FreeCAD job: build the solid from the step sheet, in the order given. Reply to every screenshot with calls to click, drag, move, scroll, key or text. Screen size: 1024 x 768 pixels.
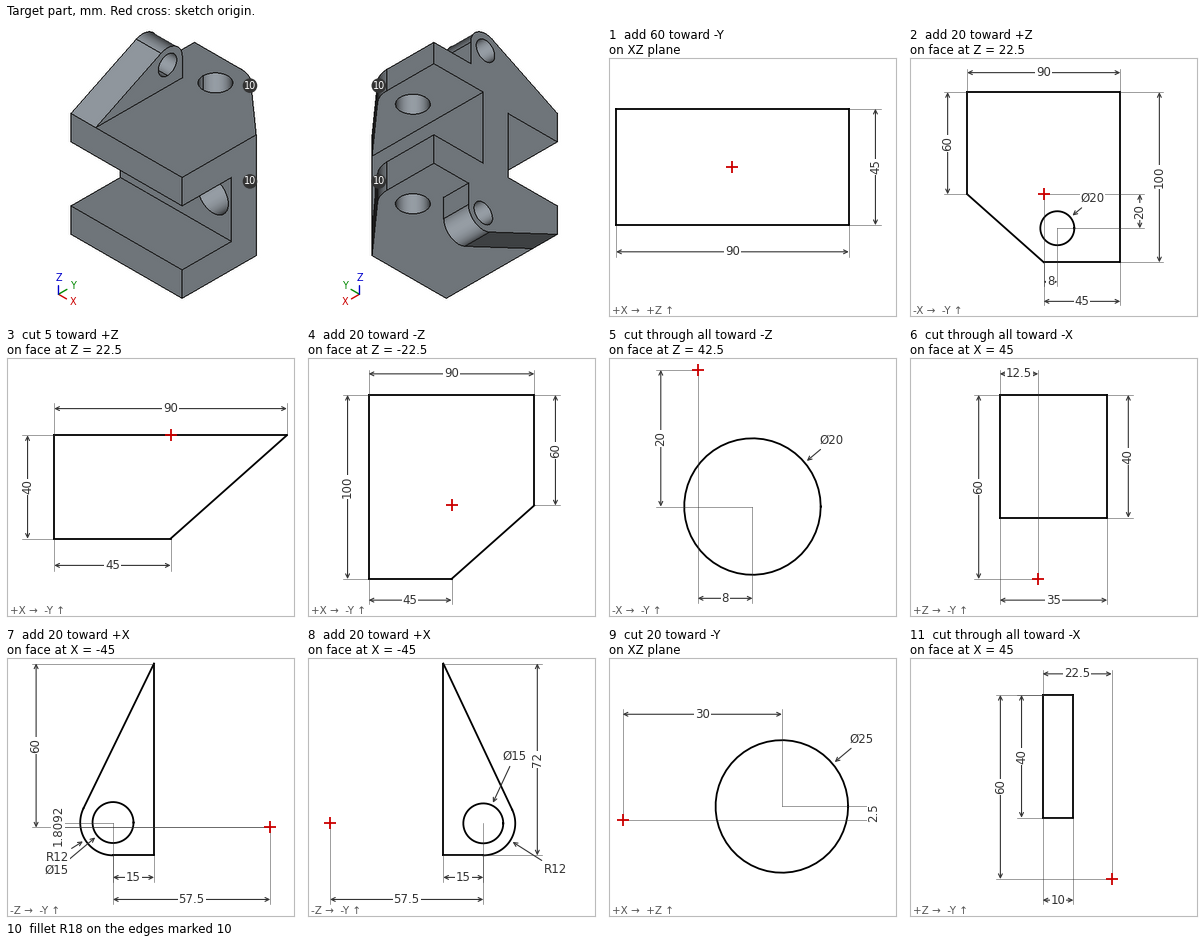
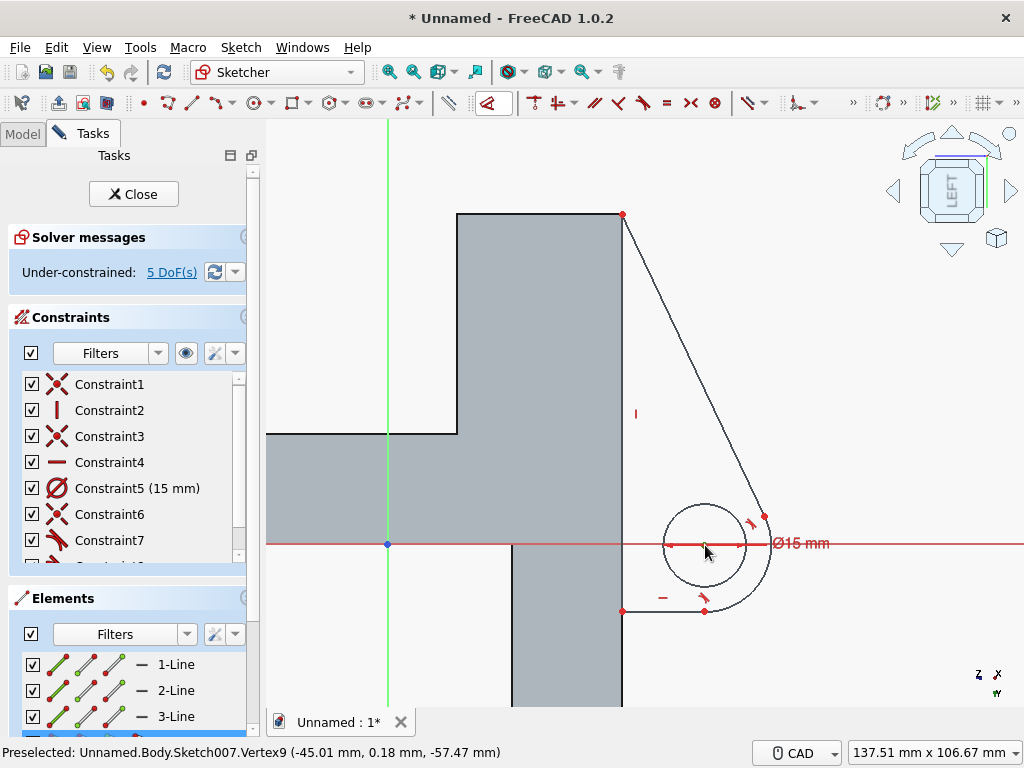
click(334, 544)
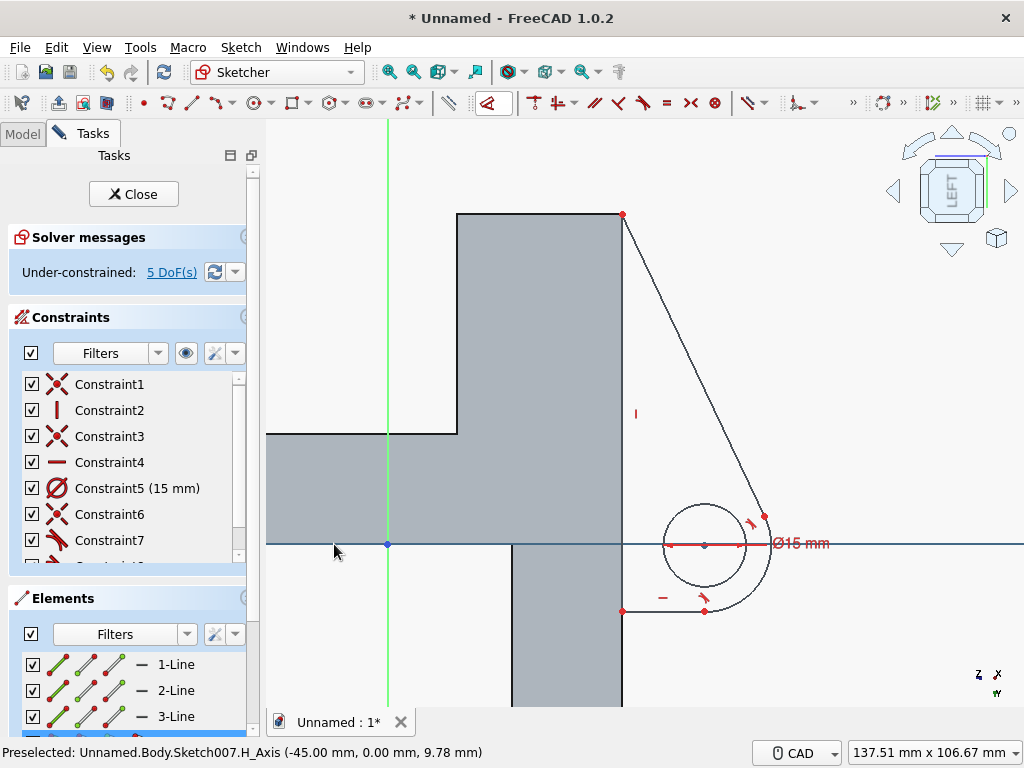
click(534, 104)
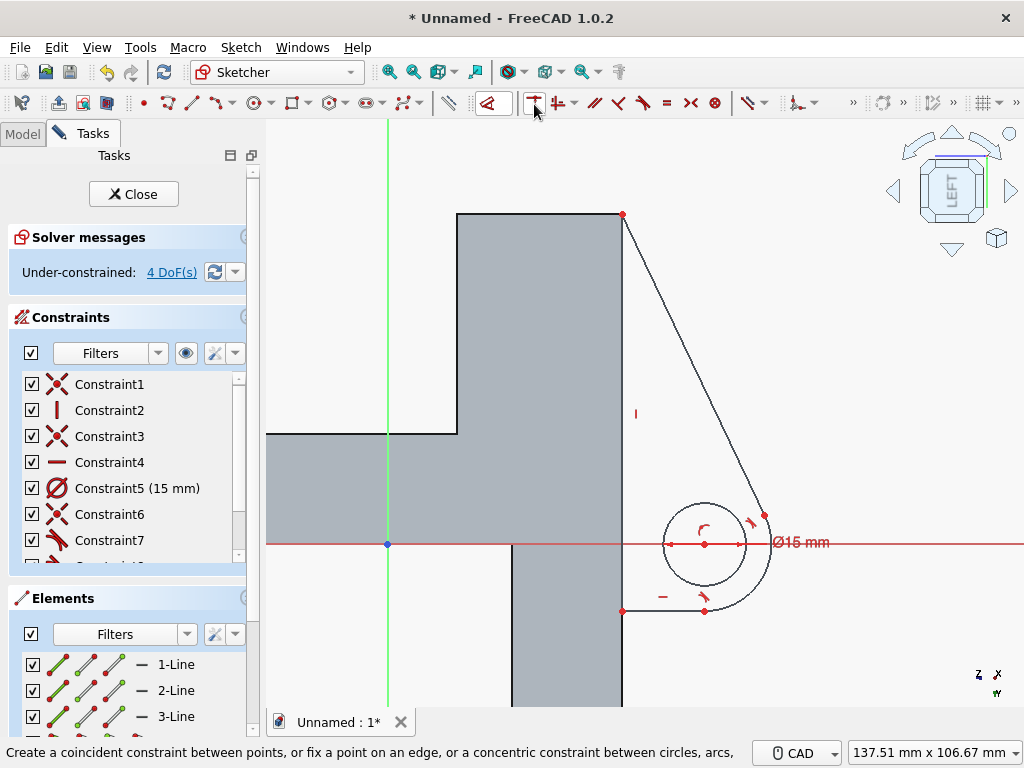
click(743, 599)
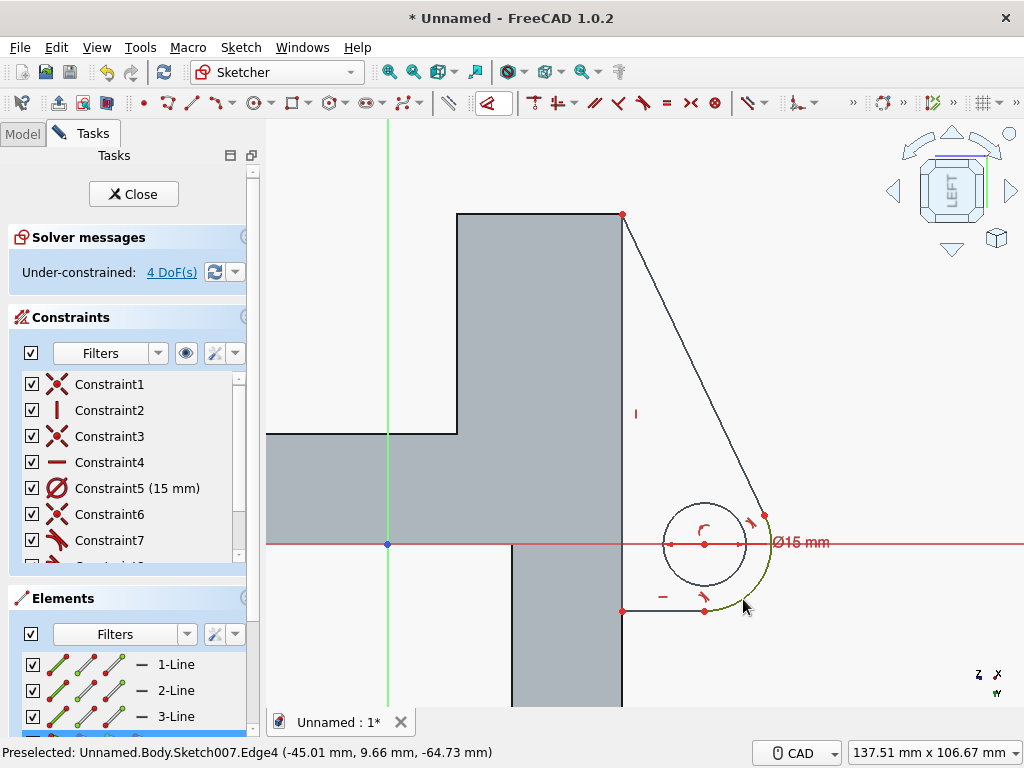
key(k)
key(r)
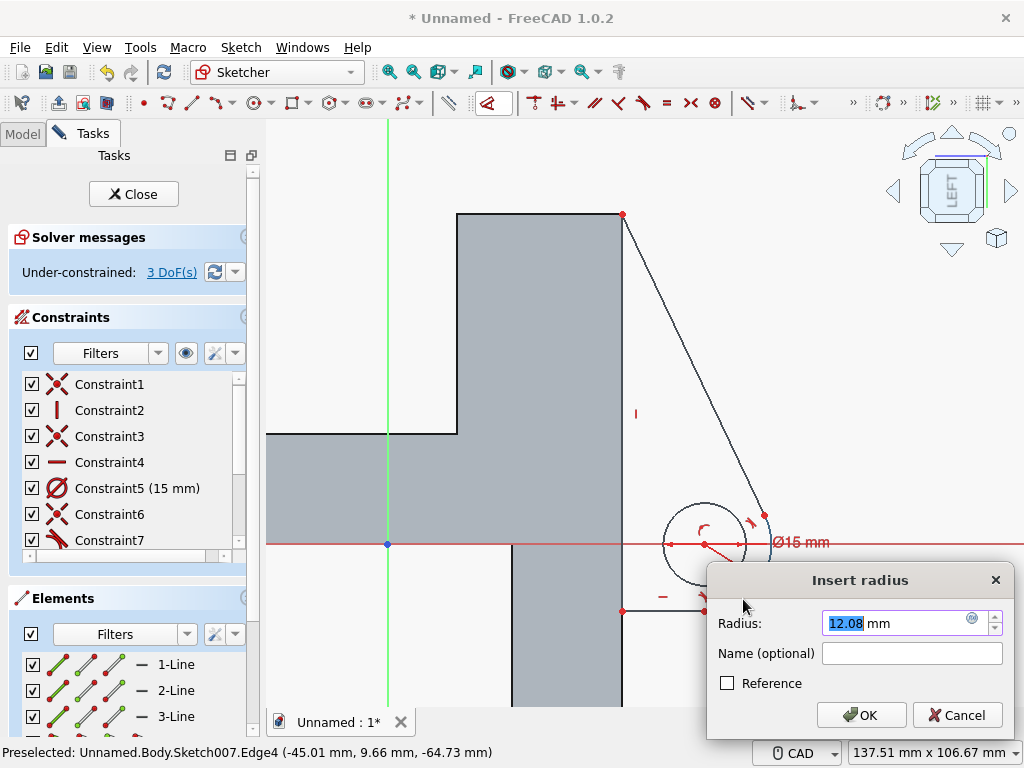
text(12)
key(Return)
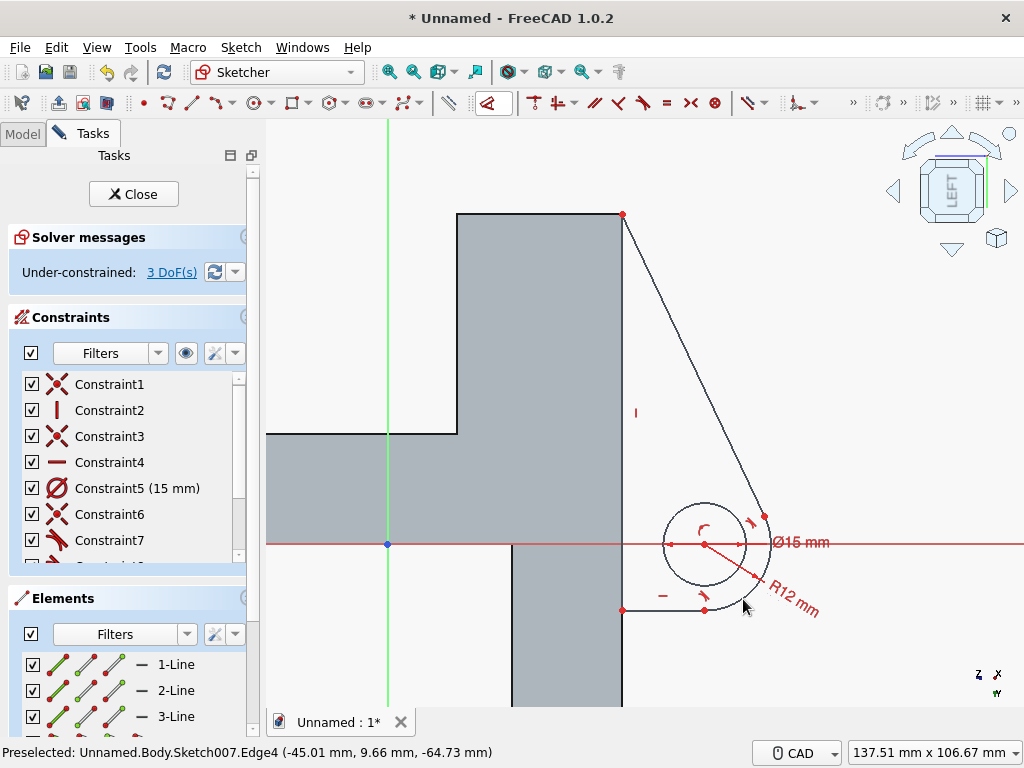
click(622, 334)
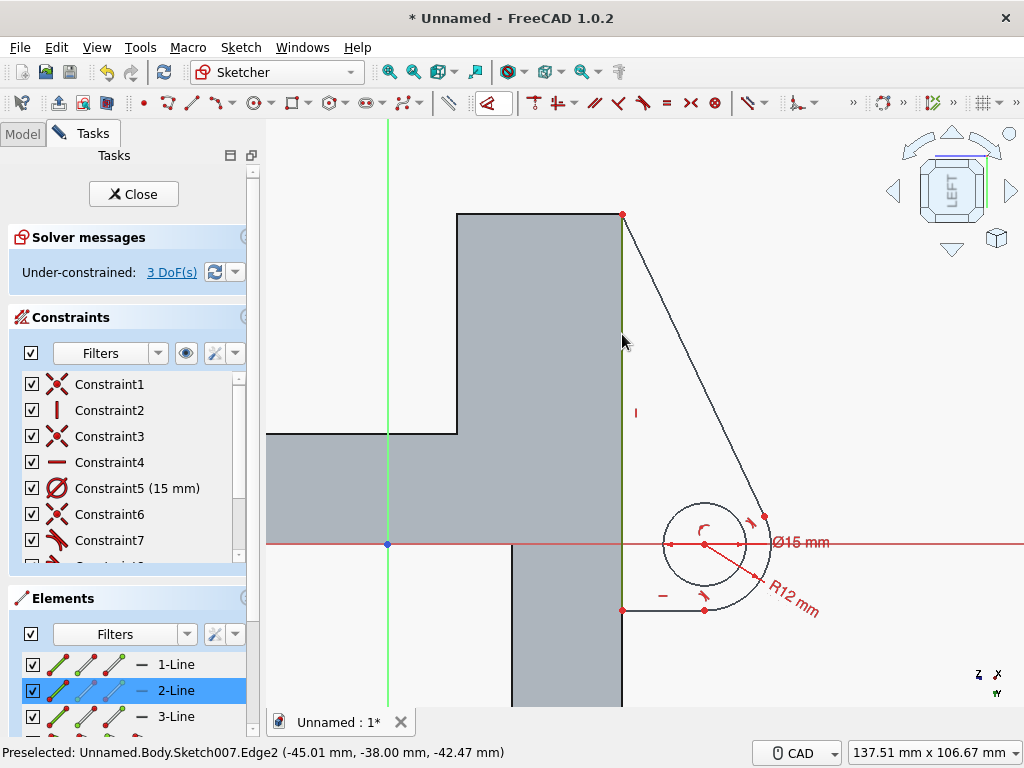
key(i)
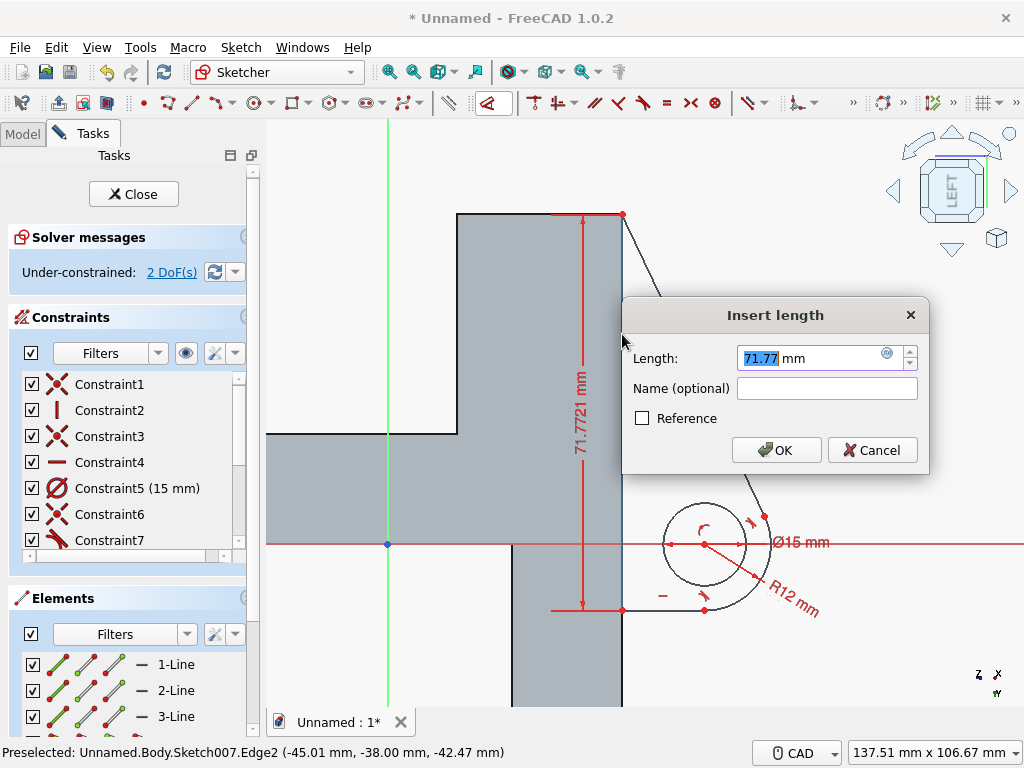
text(72)
key(Return)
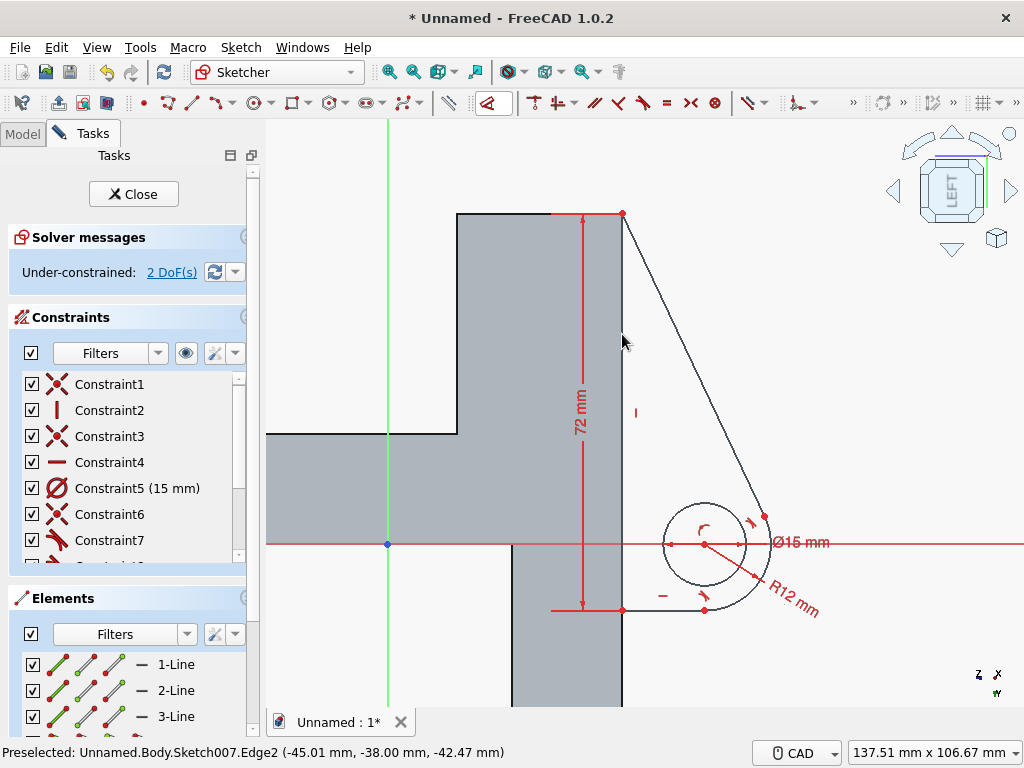
click(647, 611)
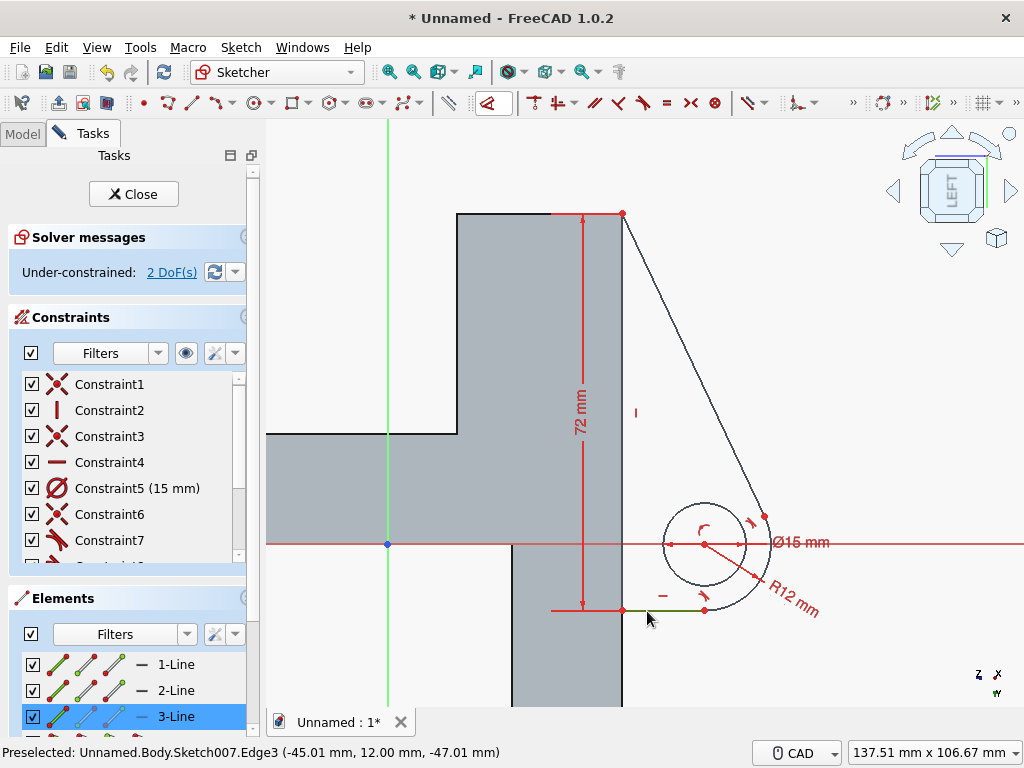
key(l)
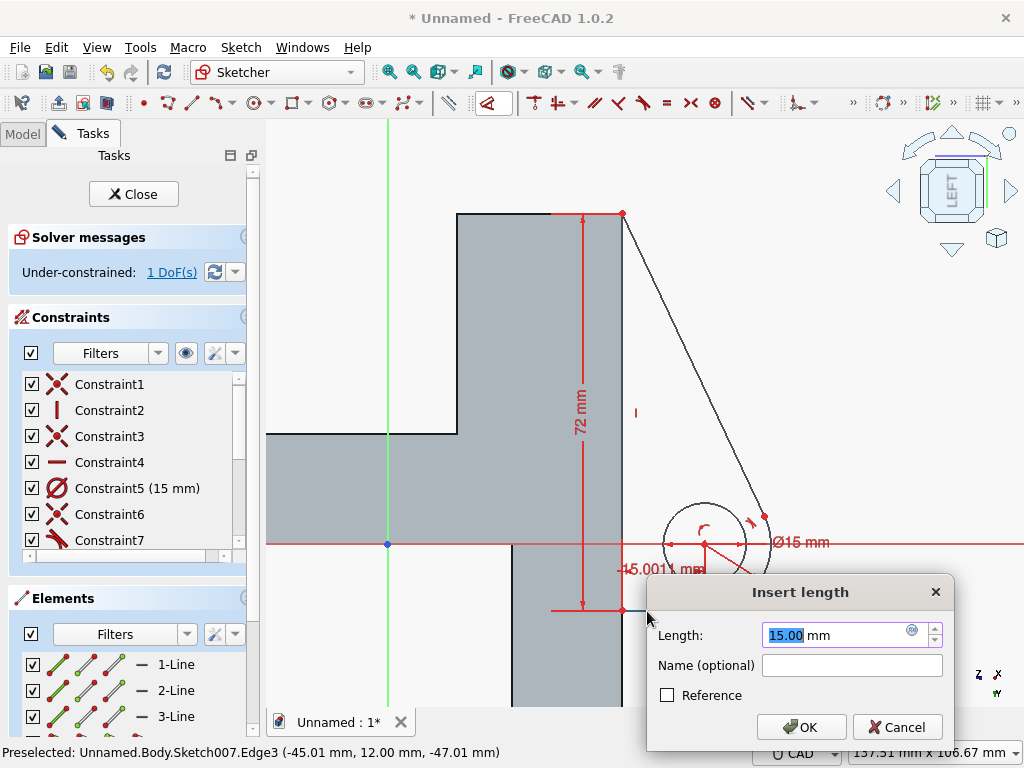
text(15)
key(Return)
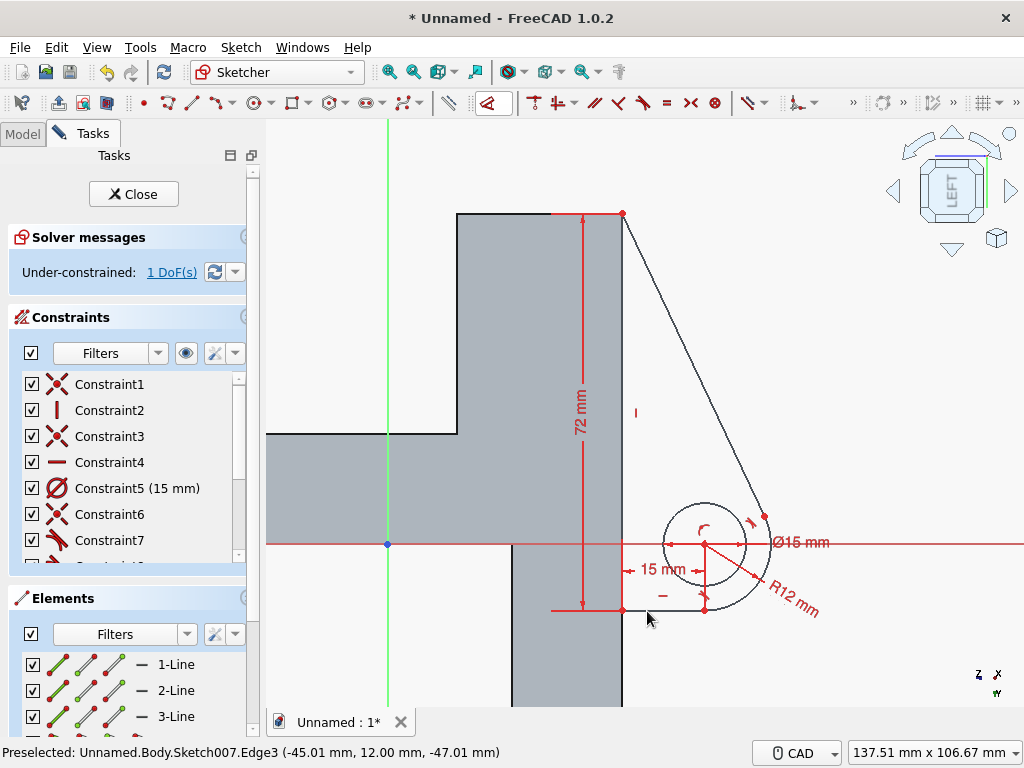
click(705, 544)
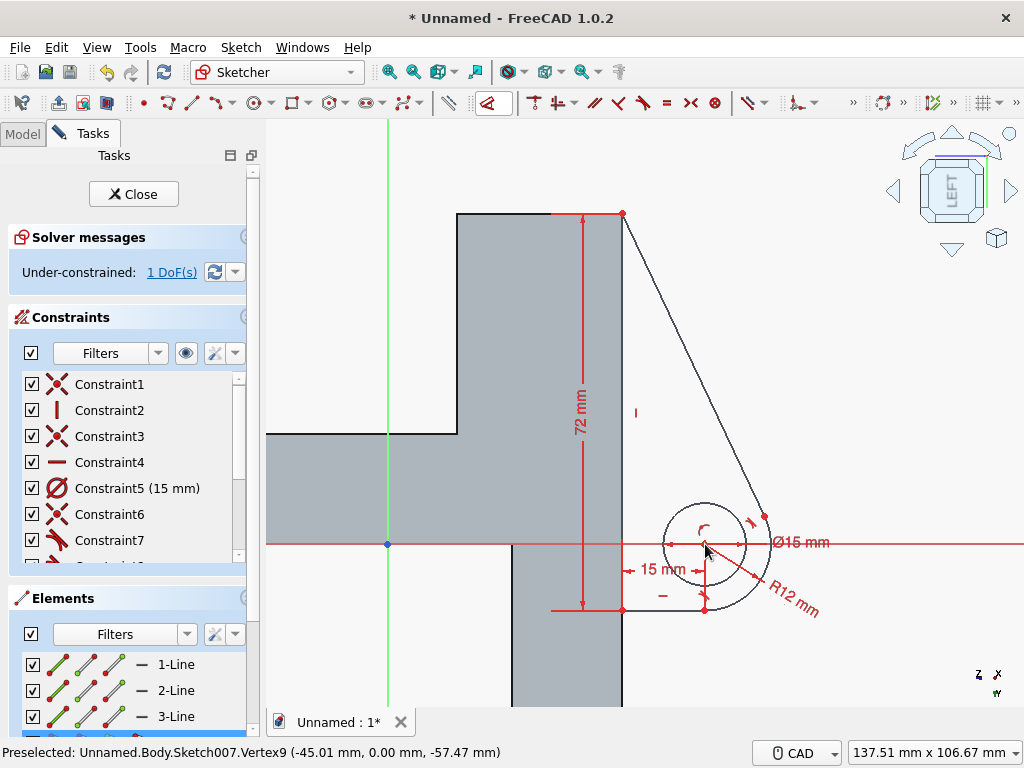
key(l)